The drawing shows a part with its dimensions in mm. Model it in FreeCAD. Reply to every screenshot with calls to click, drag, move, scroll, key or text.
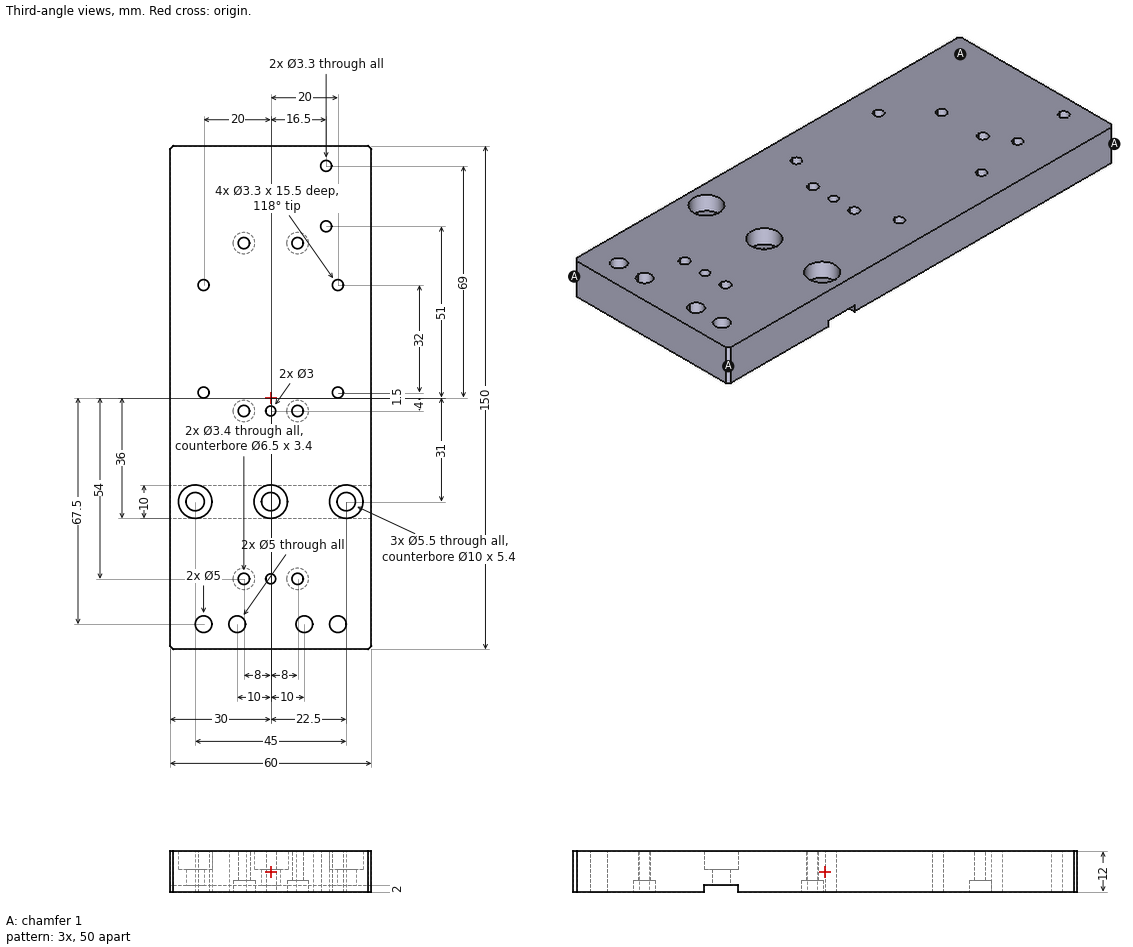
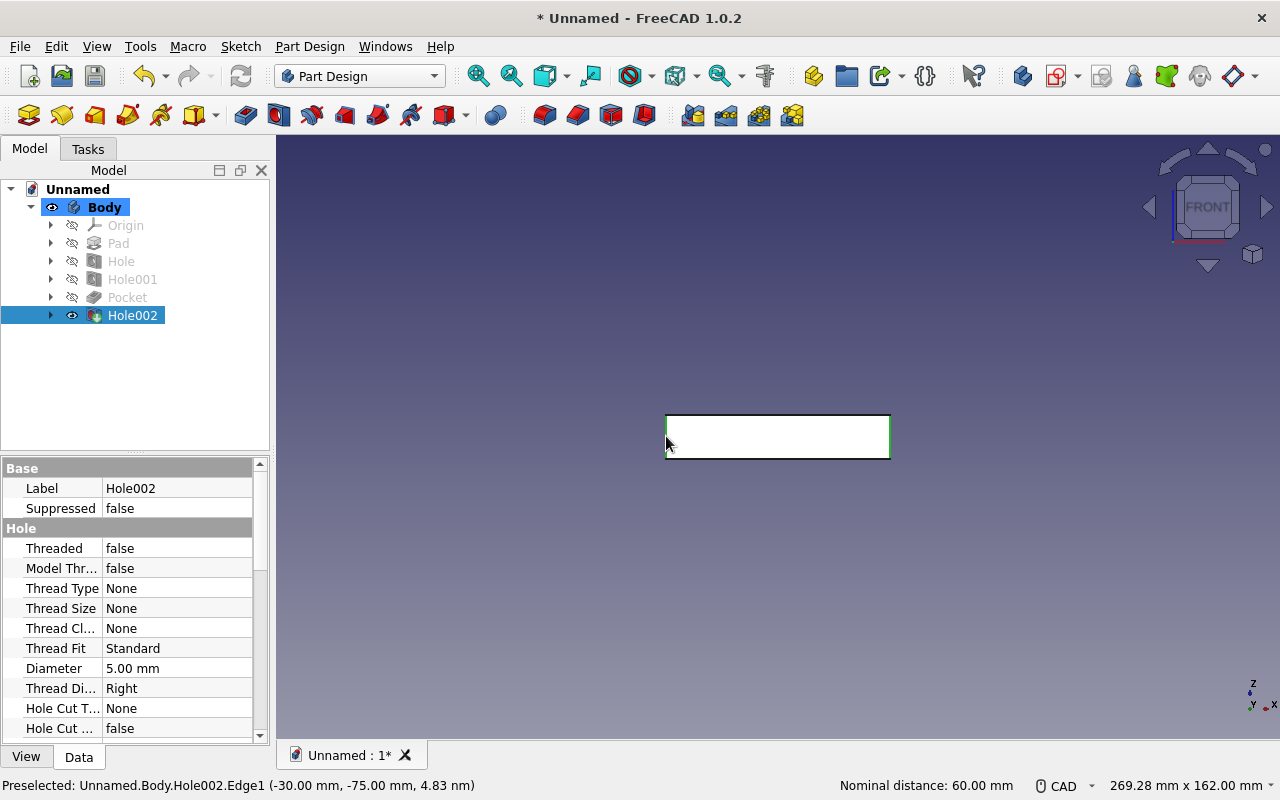
key(3)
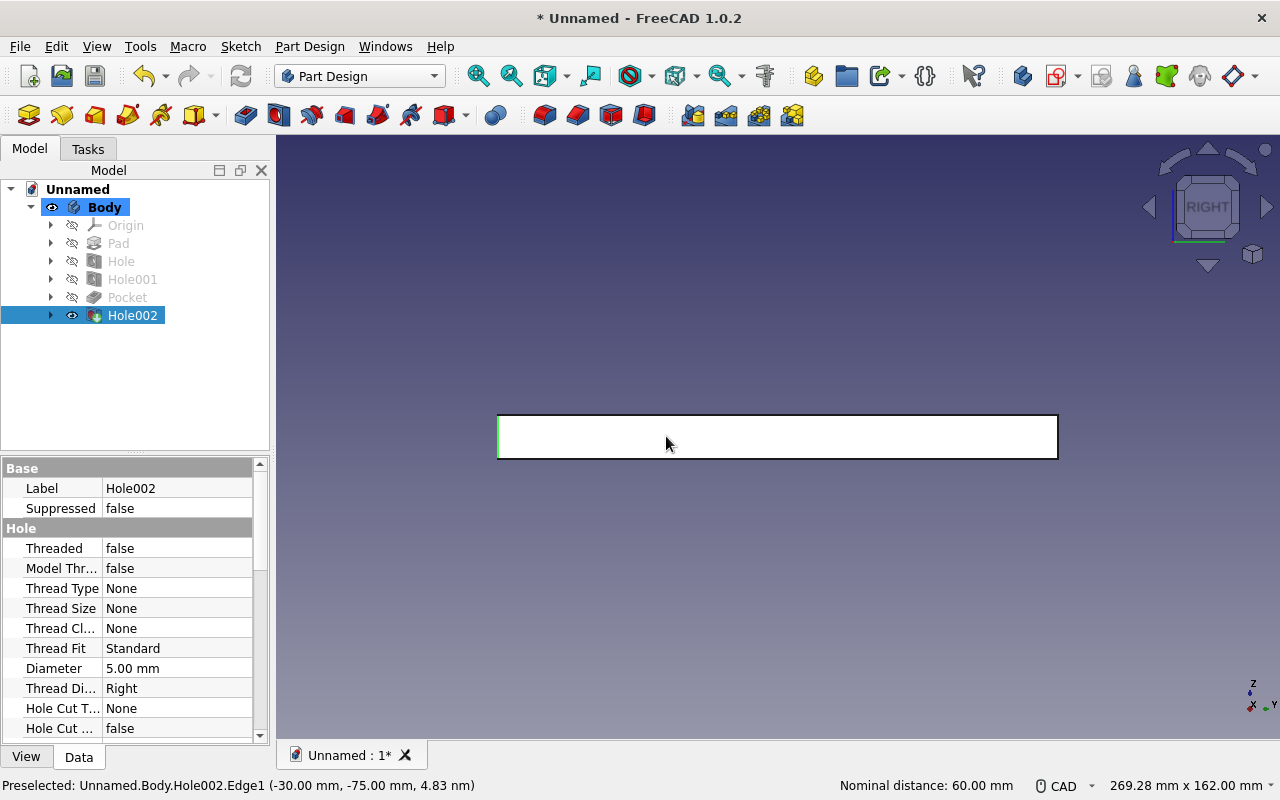
click(1058, 436, ctrl)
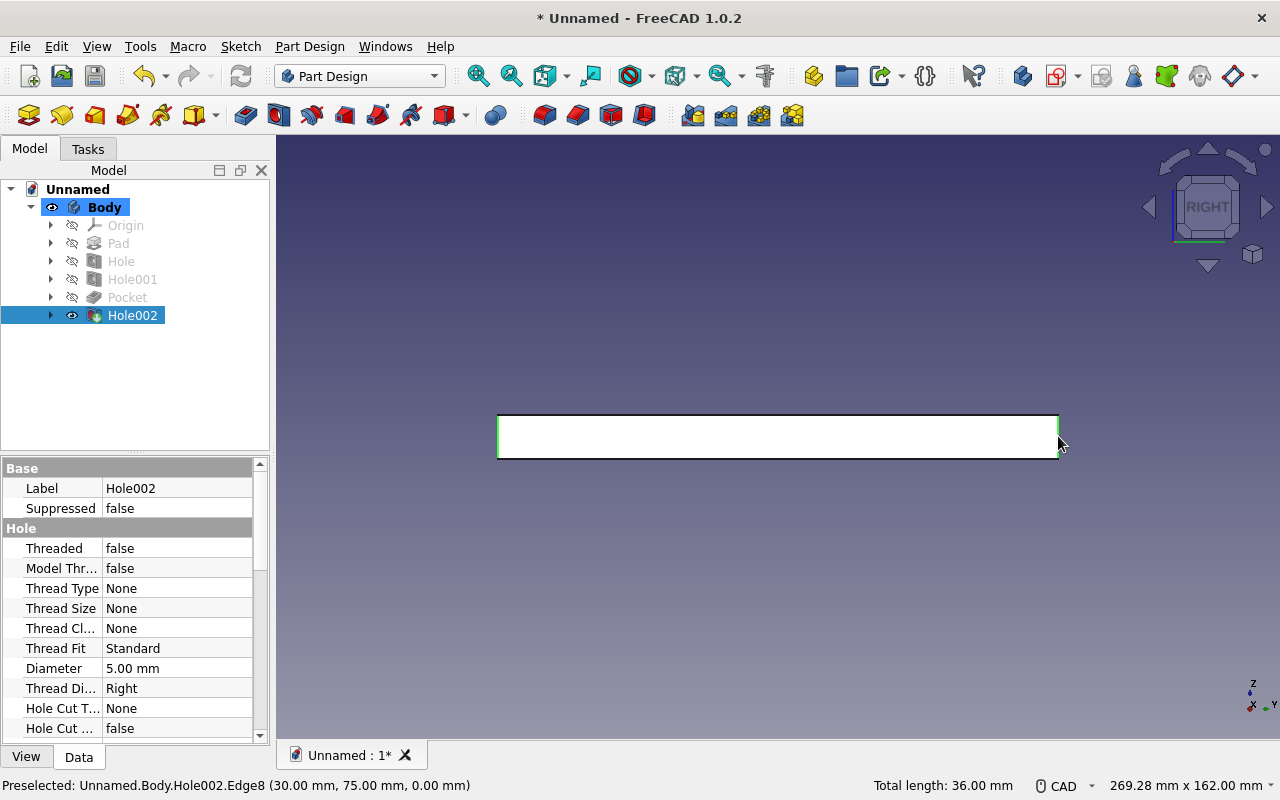
key(5)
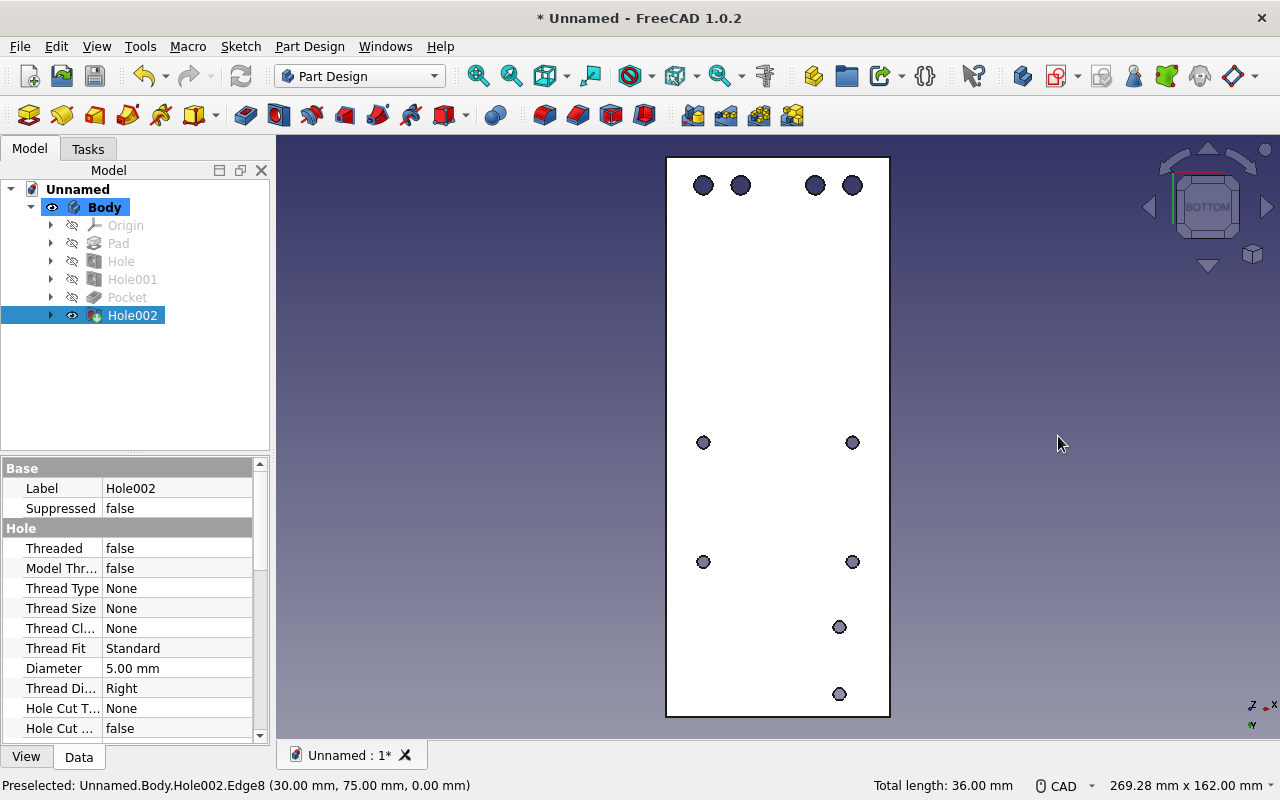
key(4)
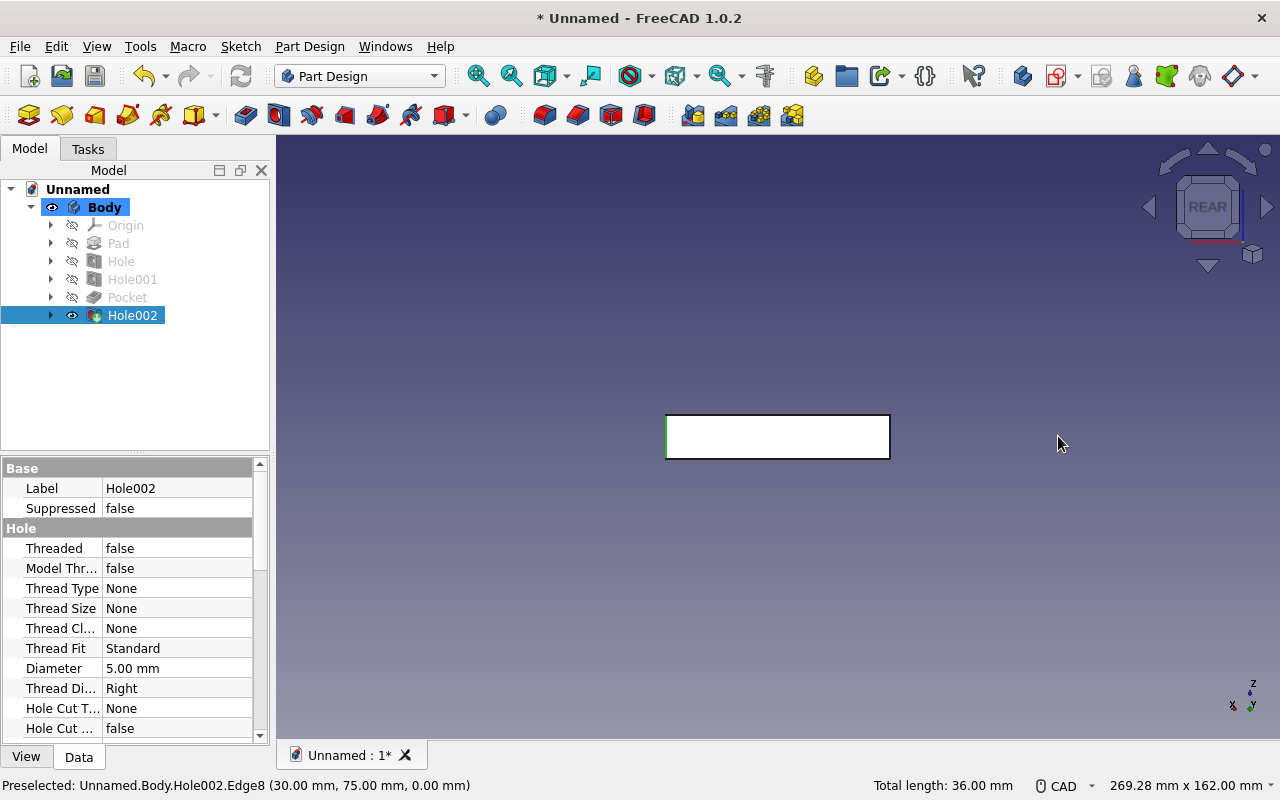
click(479, 76)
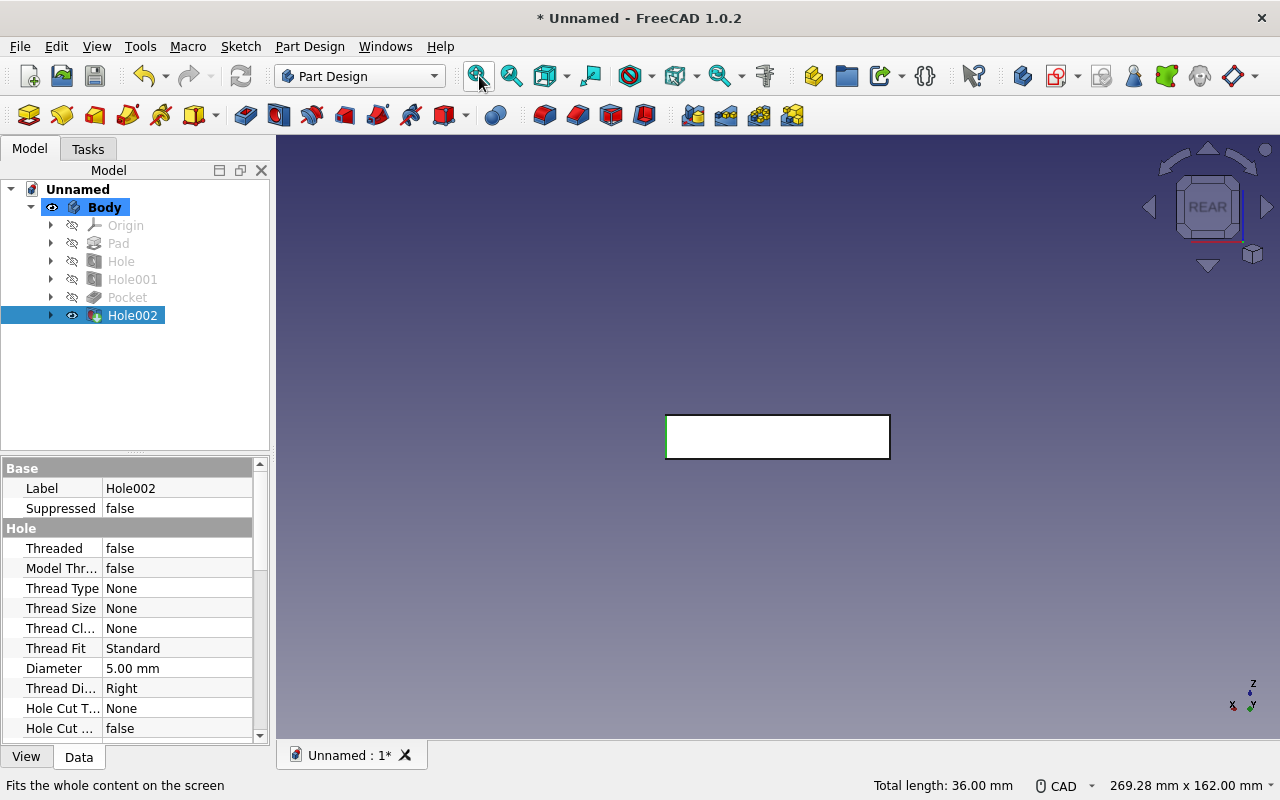
click(890, 436, ctrl)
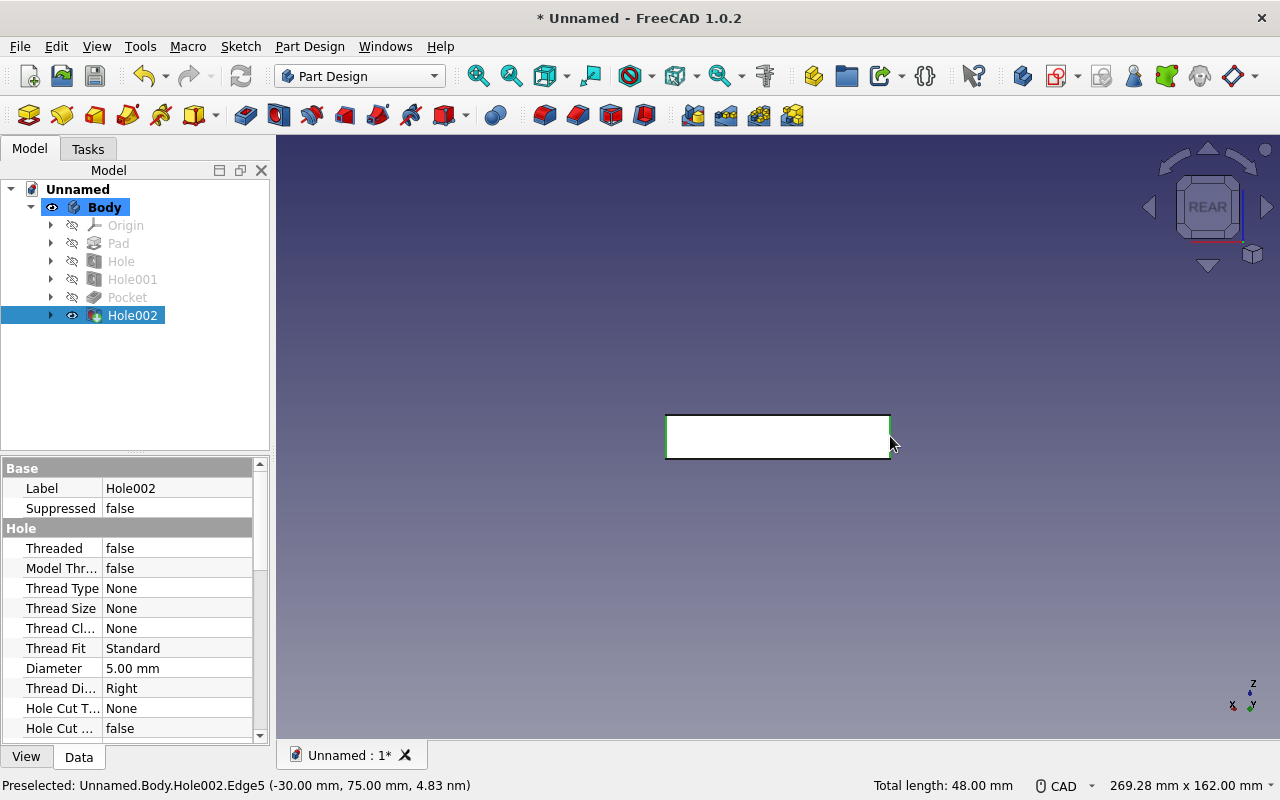
click(578, 116)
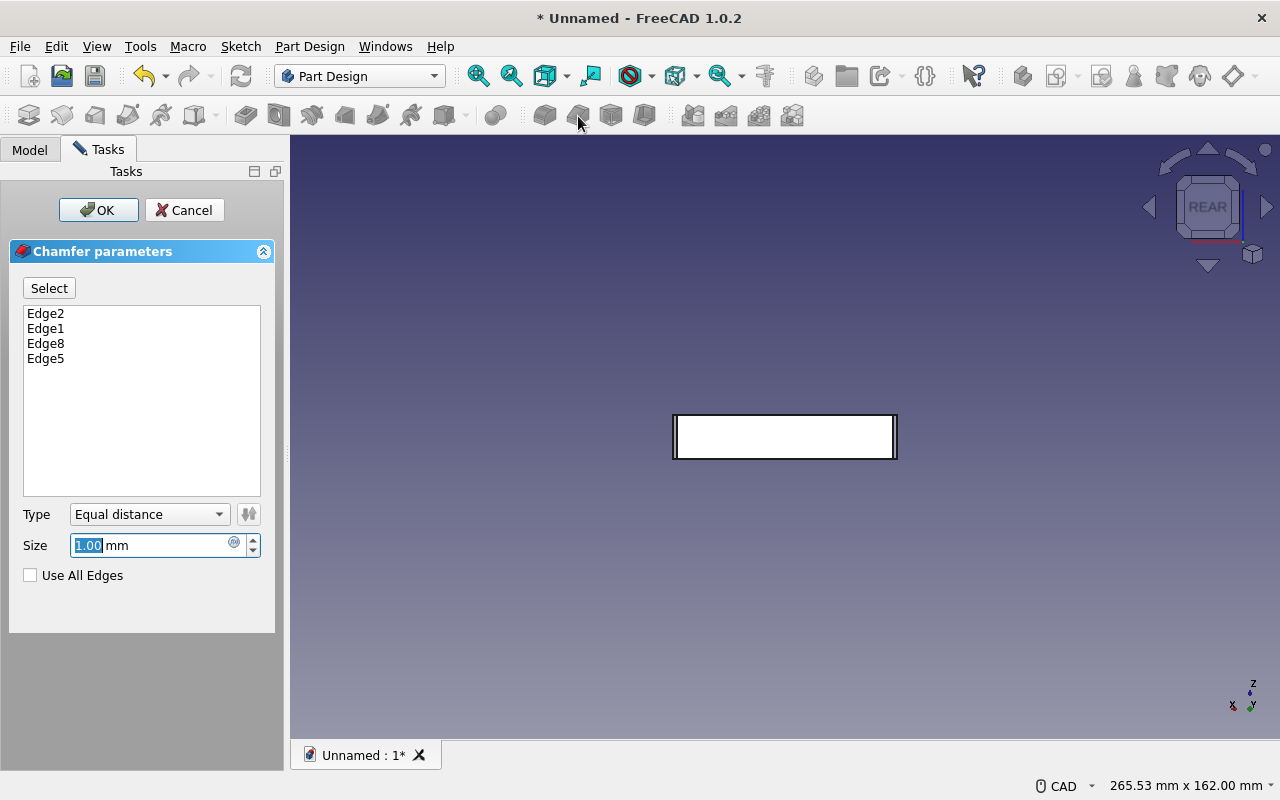
text(1)
key(Tab)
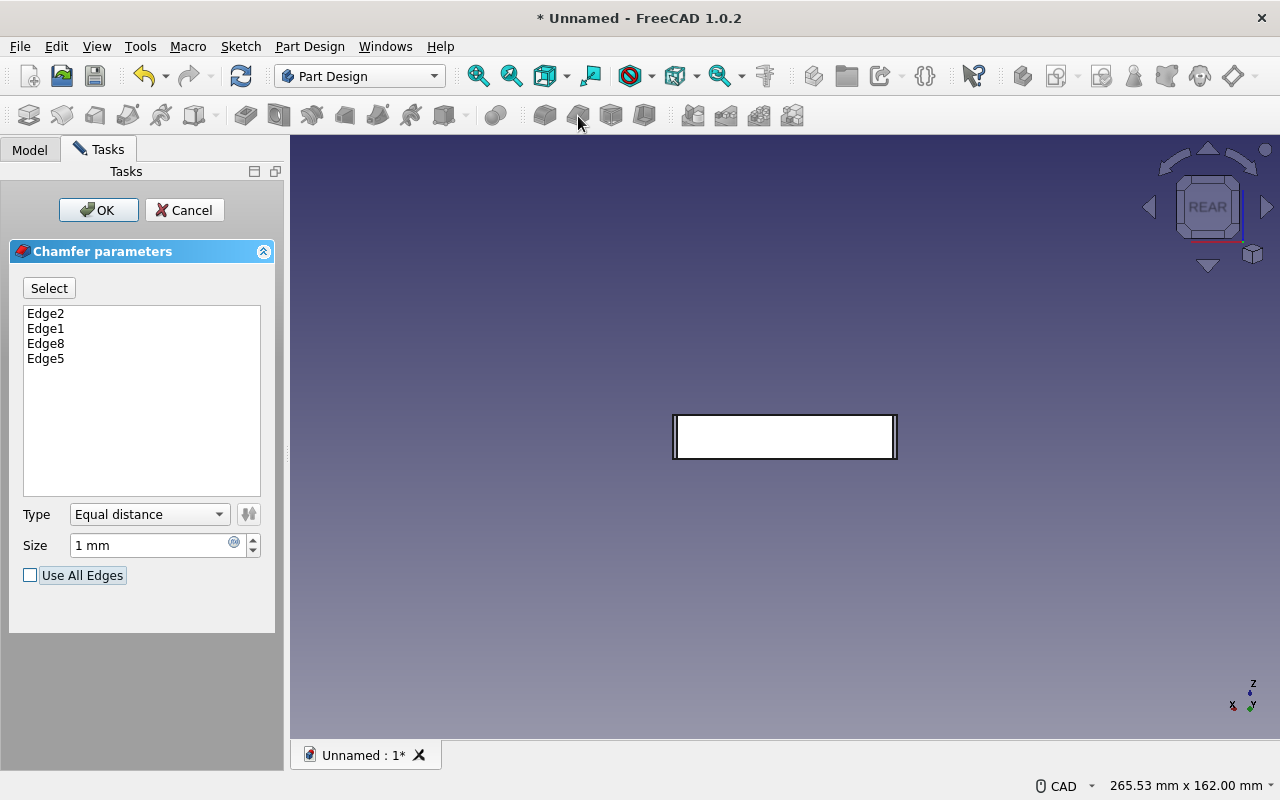
click(99, 210)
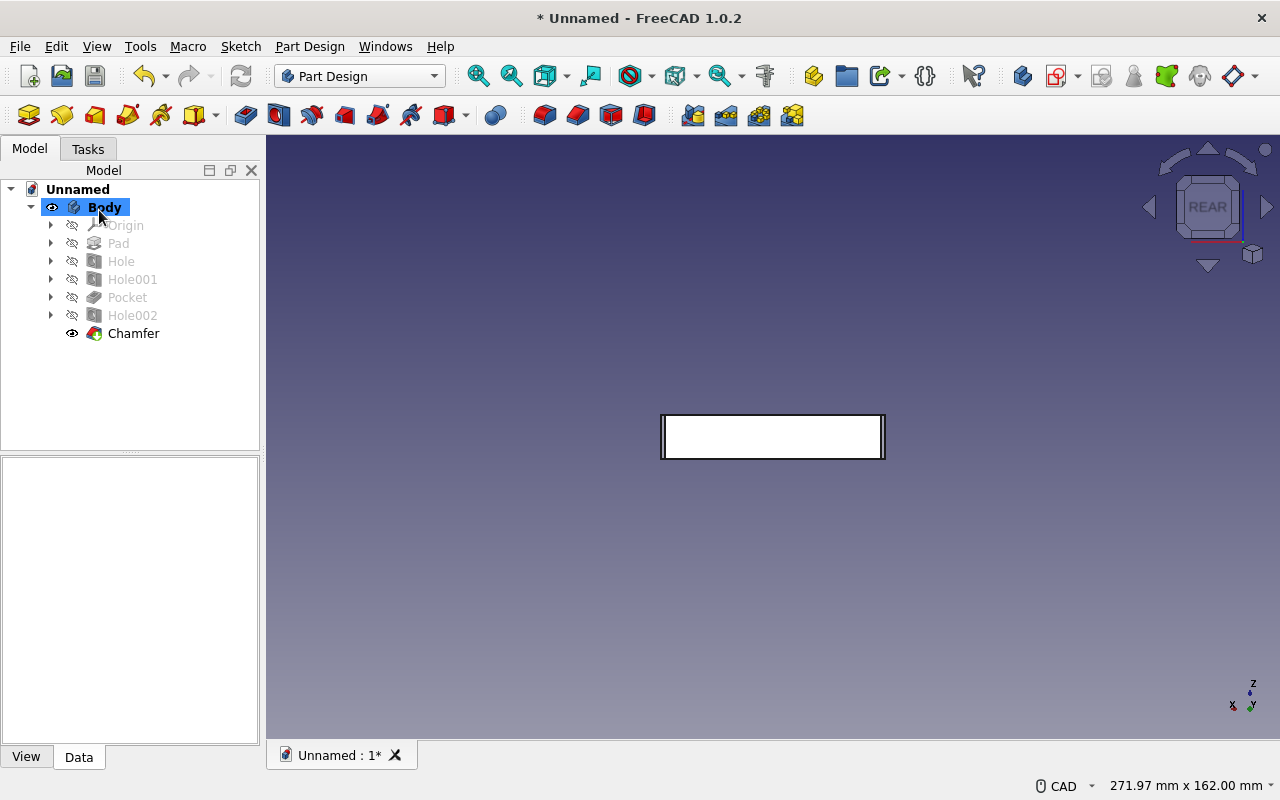
click(479, 76)